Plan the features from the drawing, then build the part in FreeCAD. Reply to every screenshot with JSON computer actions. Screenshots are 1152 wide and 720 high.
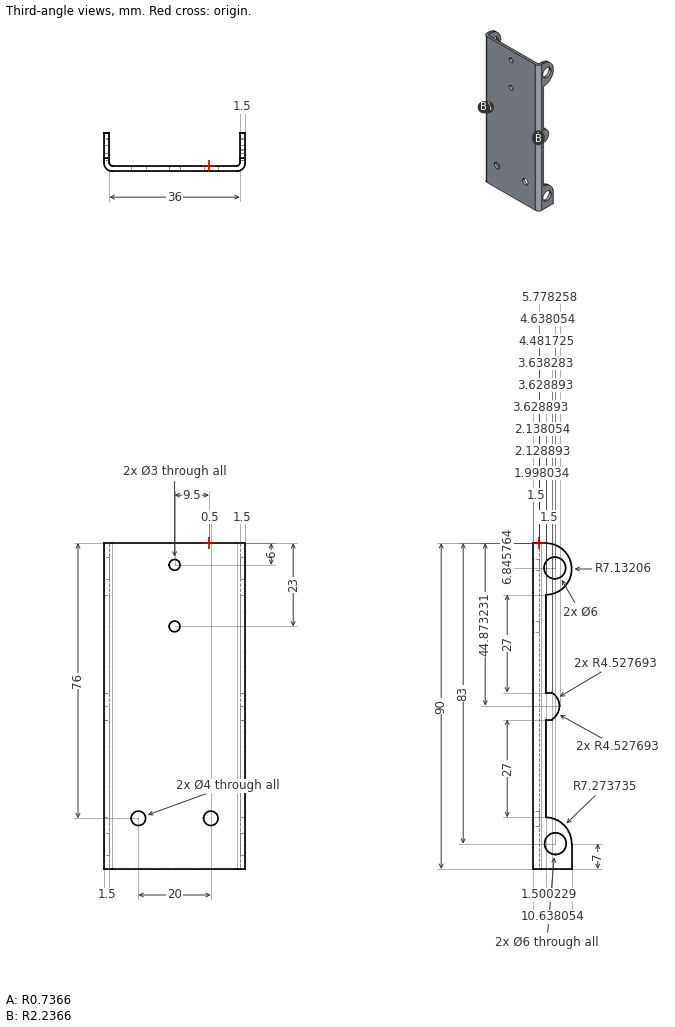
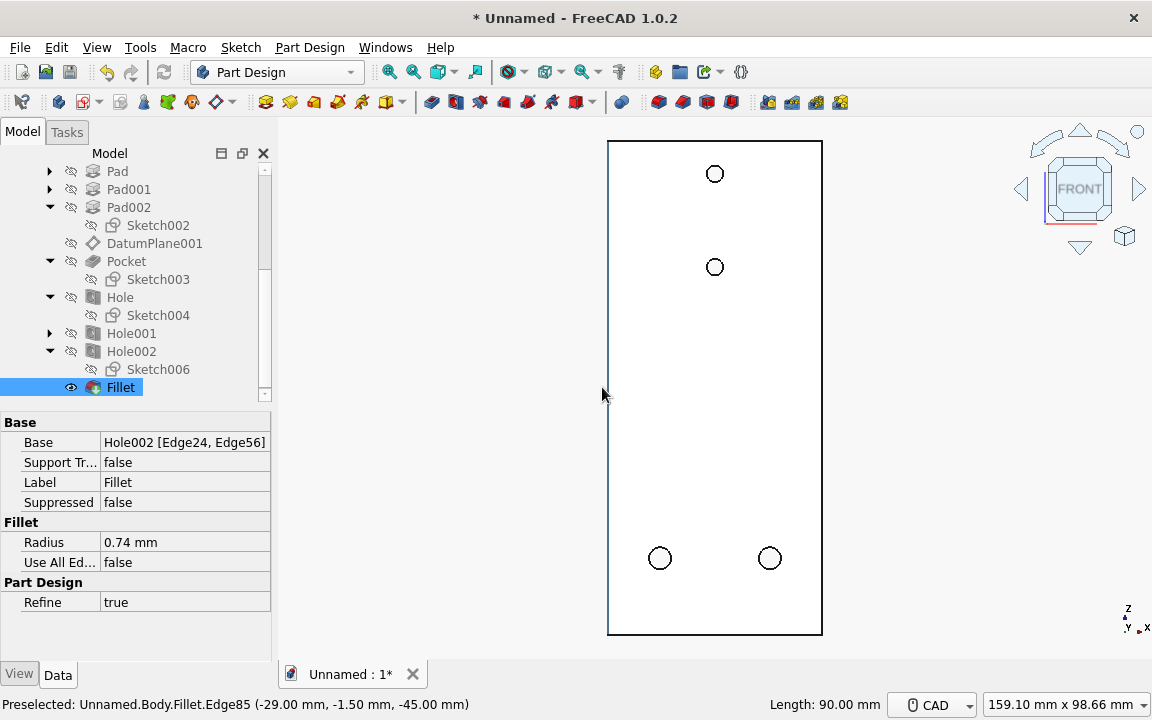
{"action": "left_click", "coordinate": [822, 387], "text": "ctrl"}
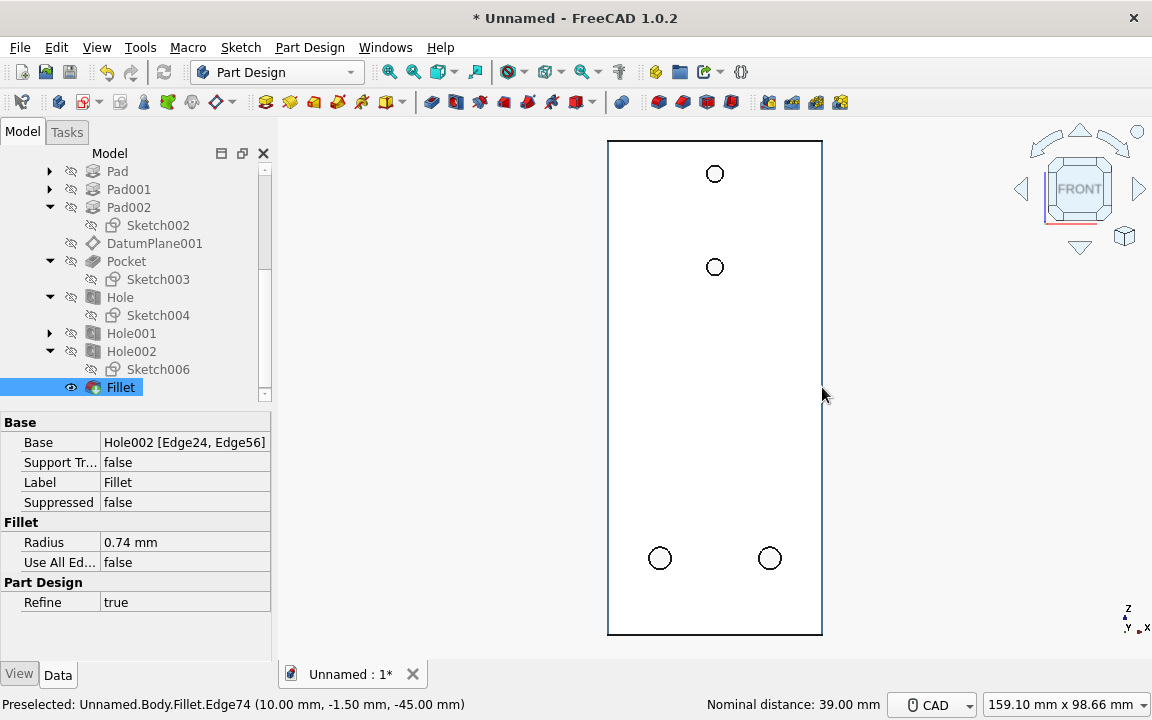
{"action": "left_click", "coordinate": [660, 102]}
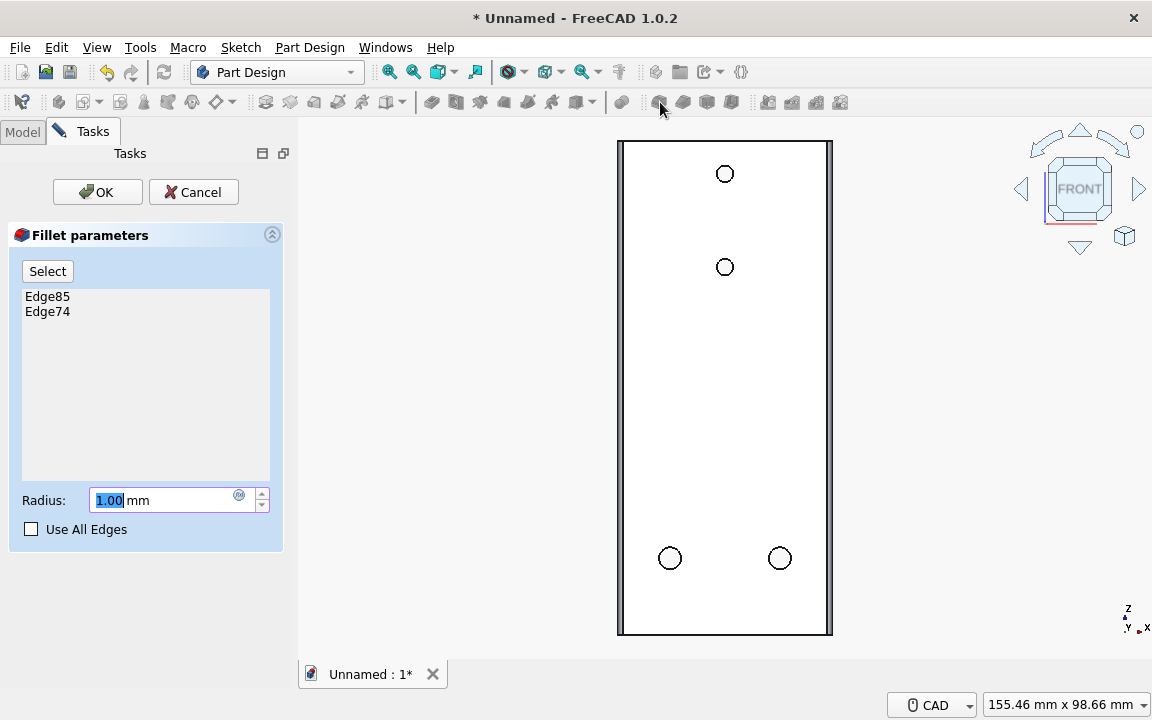
{"action": "type", "text": "2.2366"}
{"action": "key", "text": "Tab"}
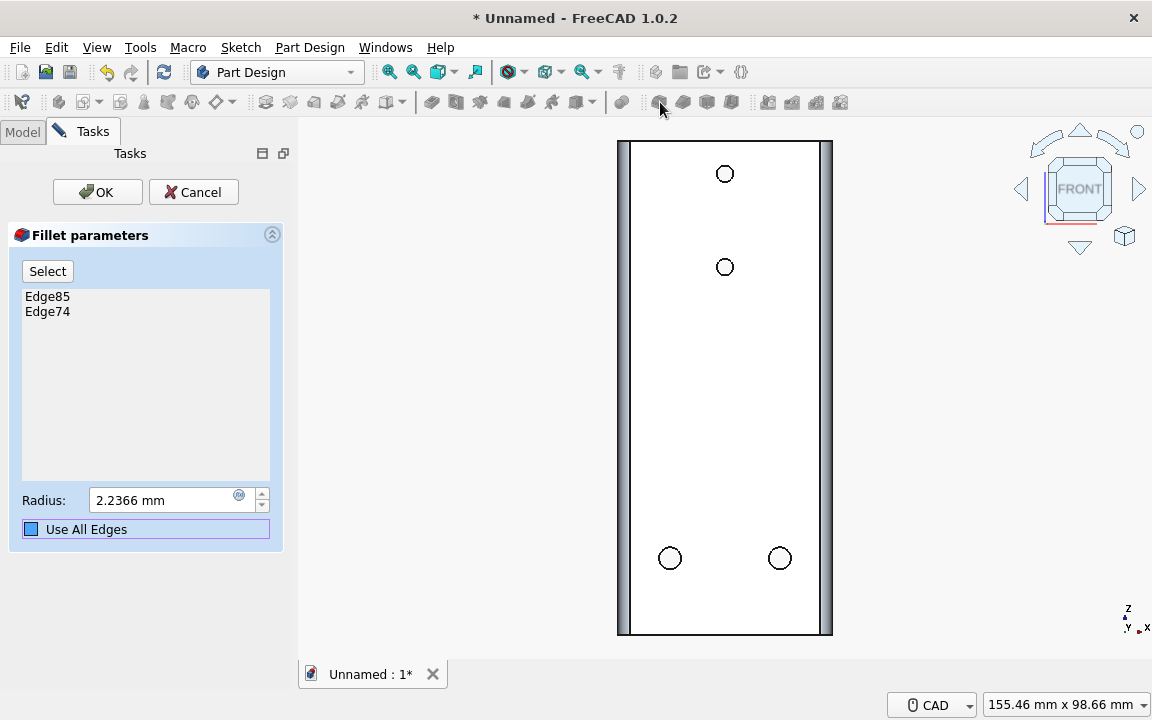
{"action": "left_click", "coordinate": [98, 192]}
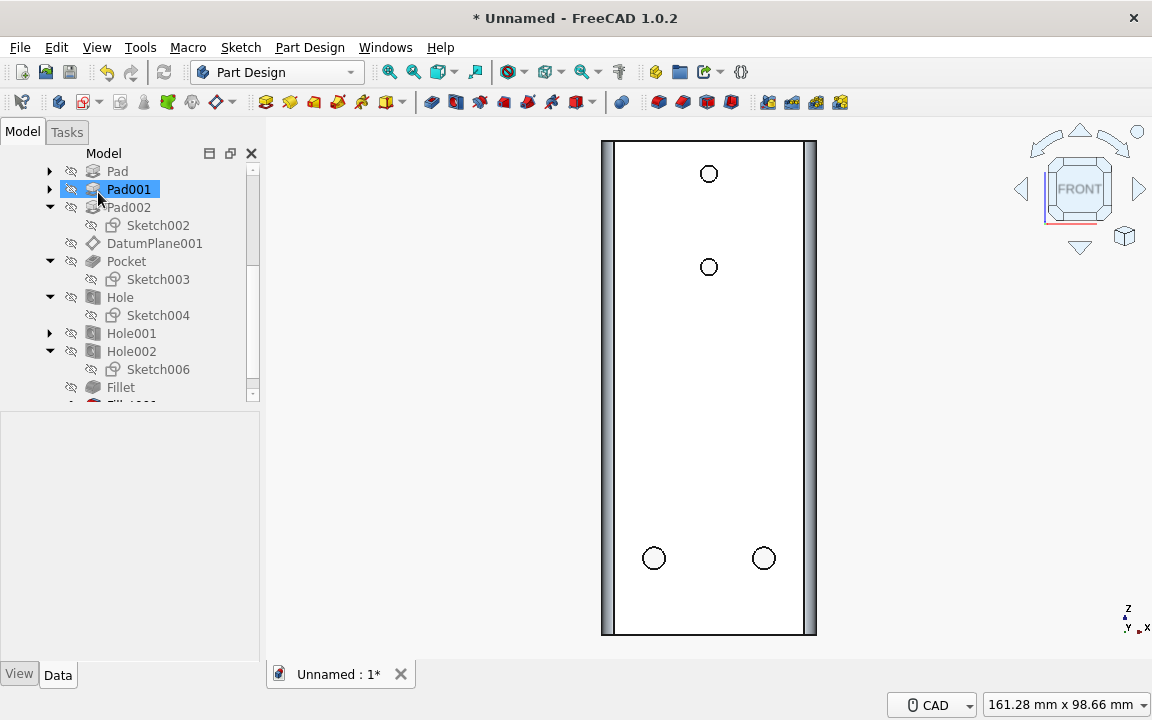
{"action": "key", "text": "0"}